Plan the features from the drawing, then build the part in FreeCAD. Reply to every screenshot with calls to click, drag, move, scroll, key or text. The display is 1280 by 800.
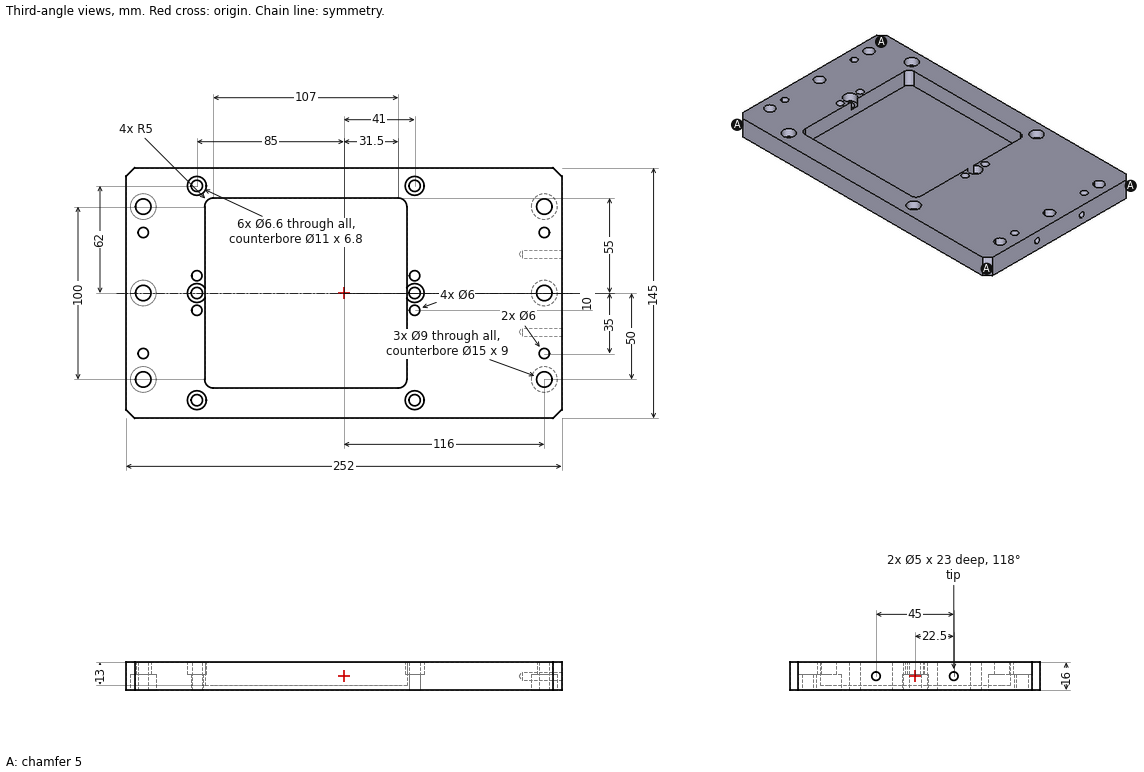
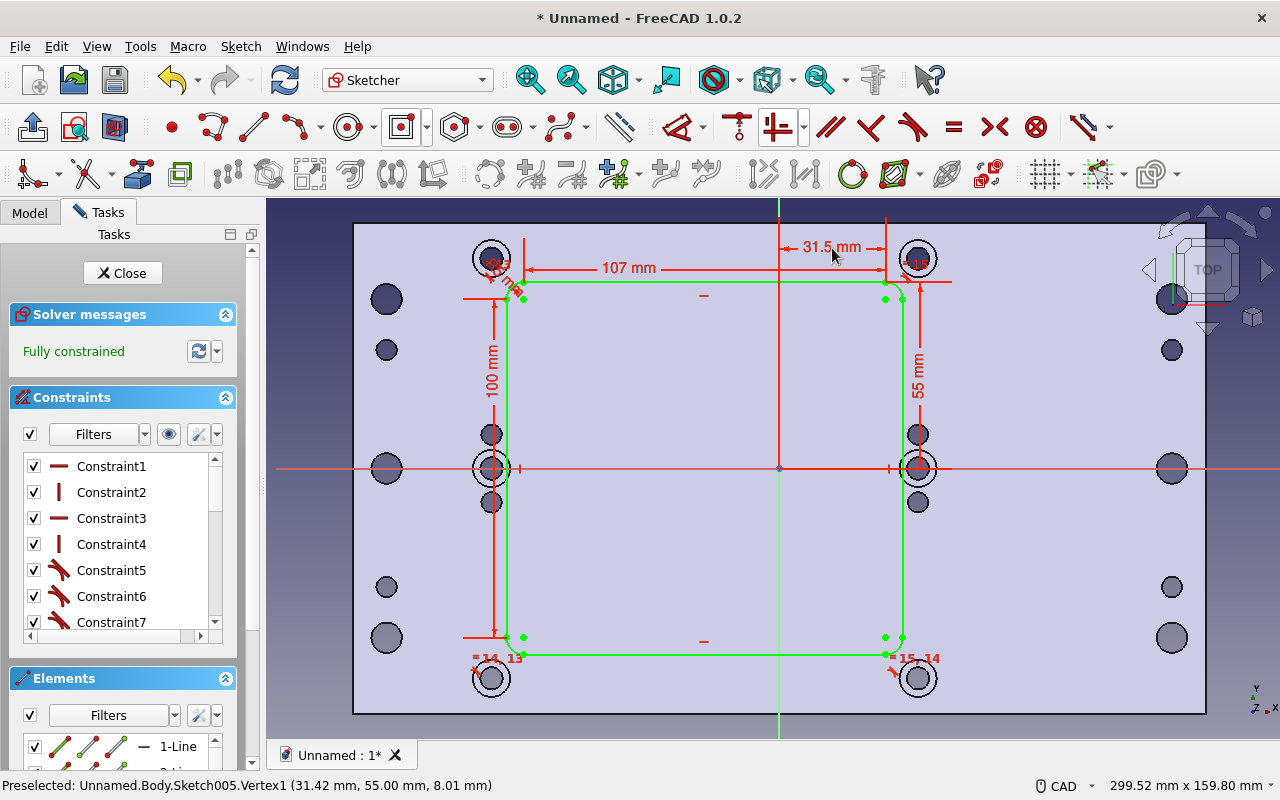
click(123, 273)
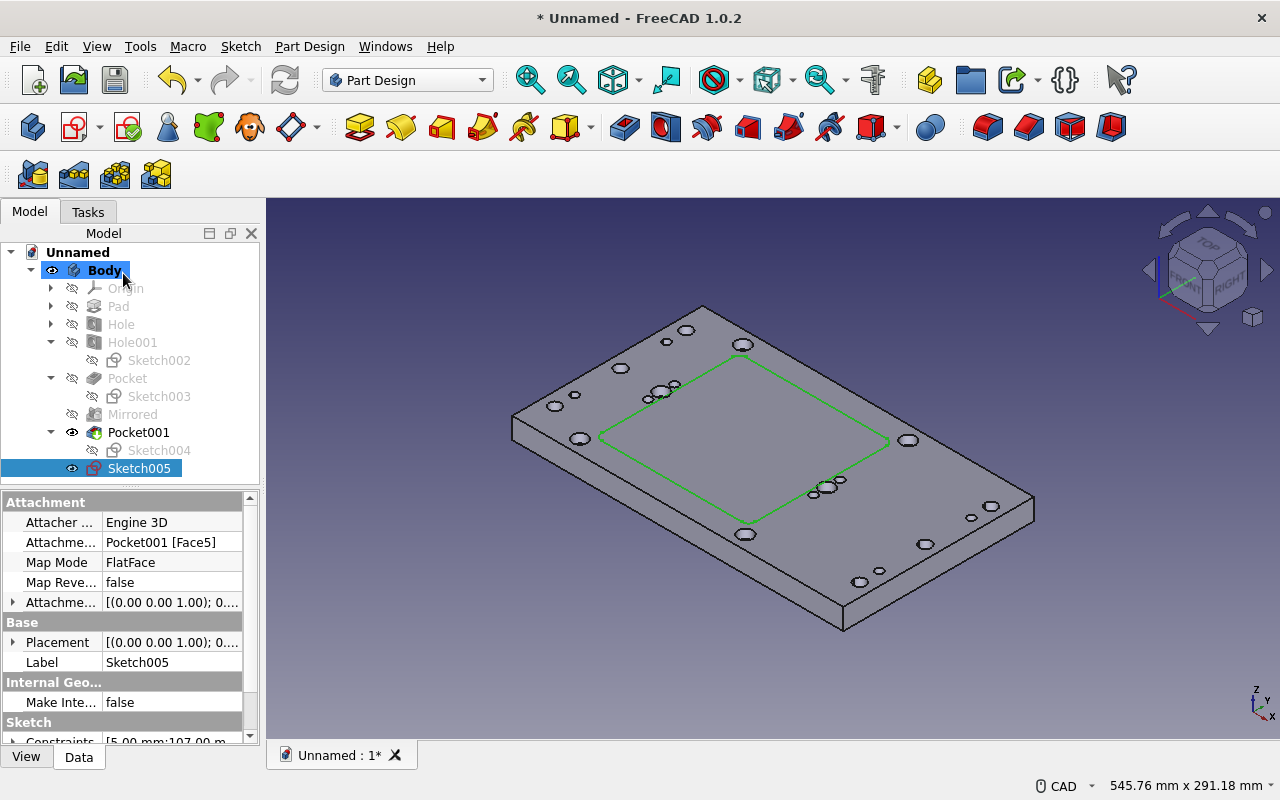
click(625, 128)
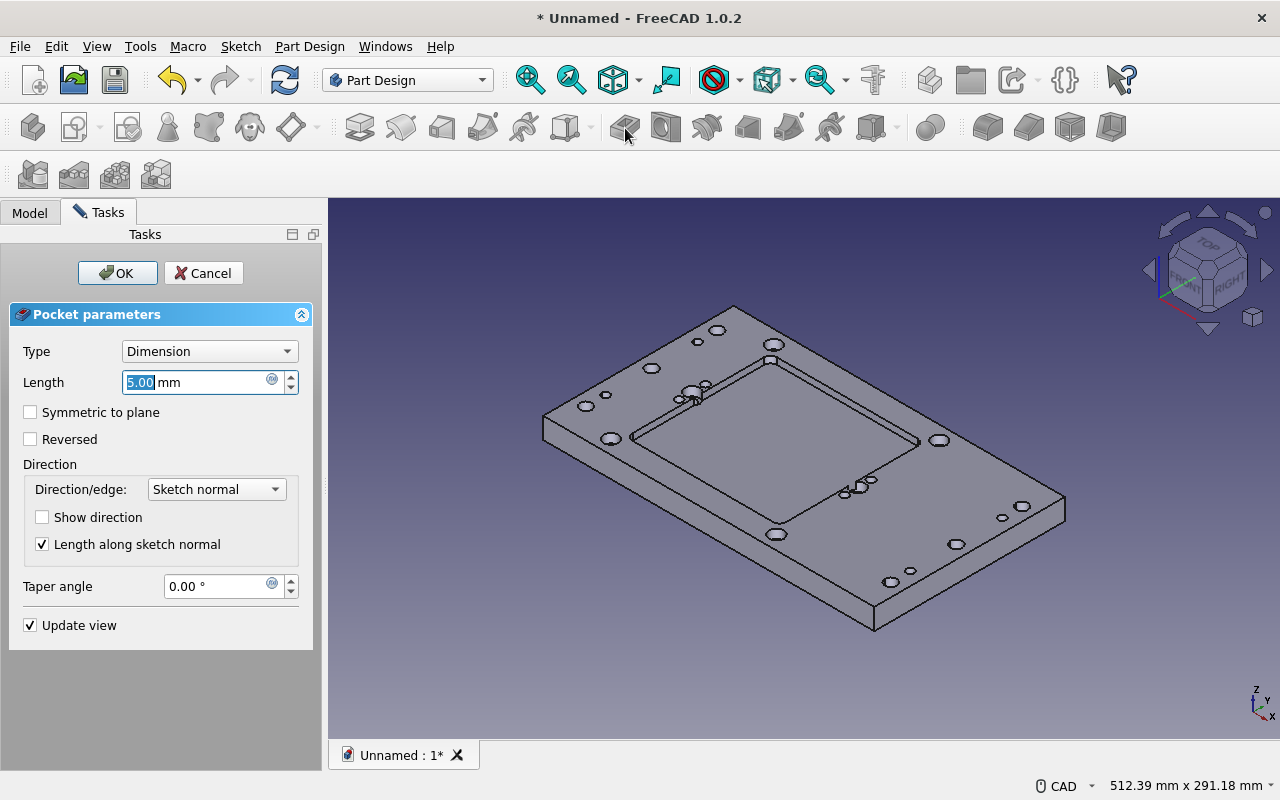
text(13)
key(Tab)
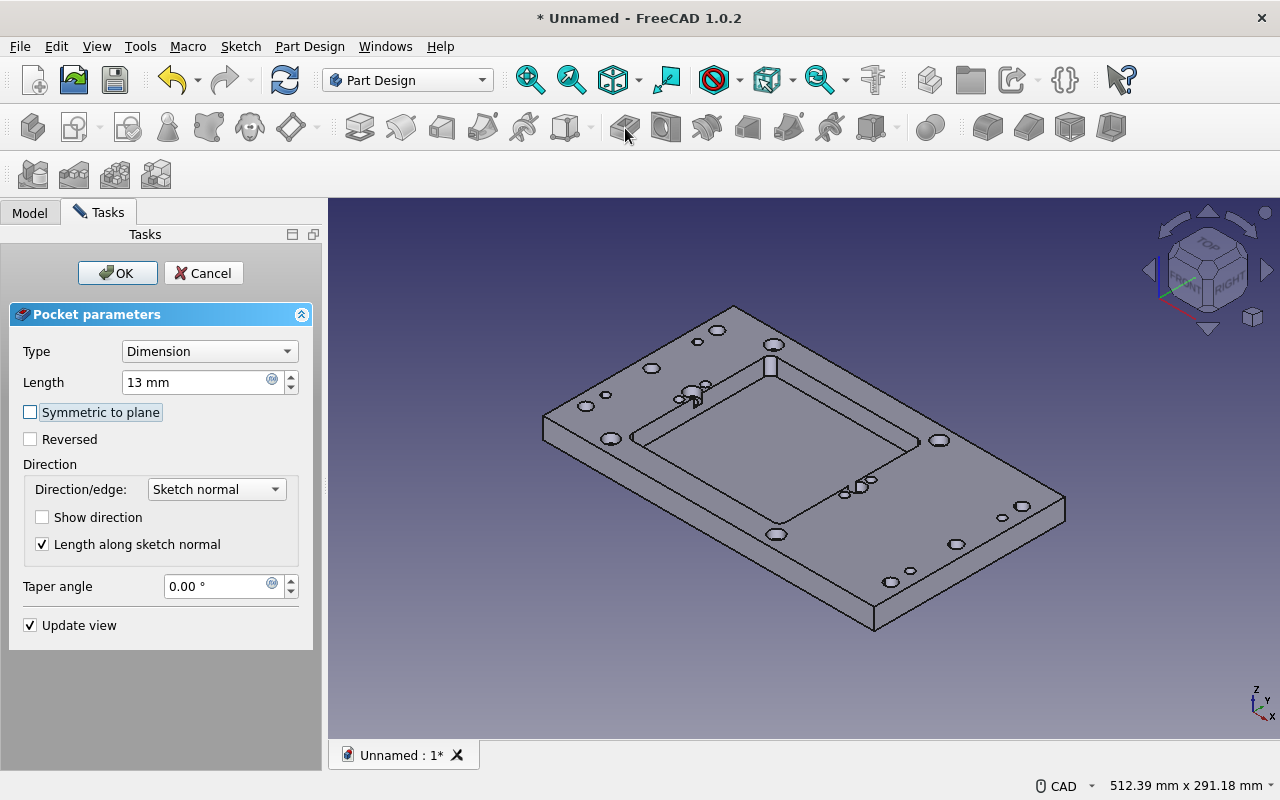
click(118, 273)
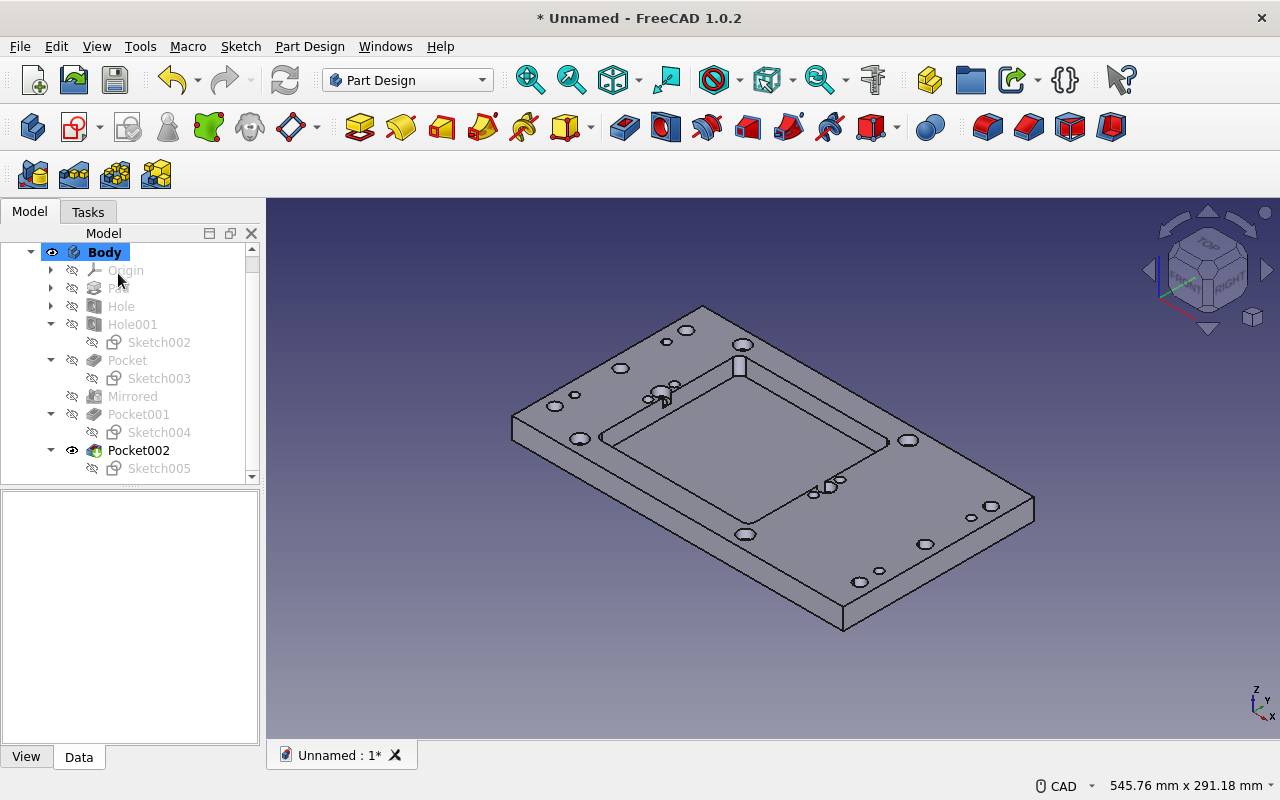
click(843, 618)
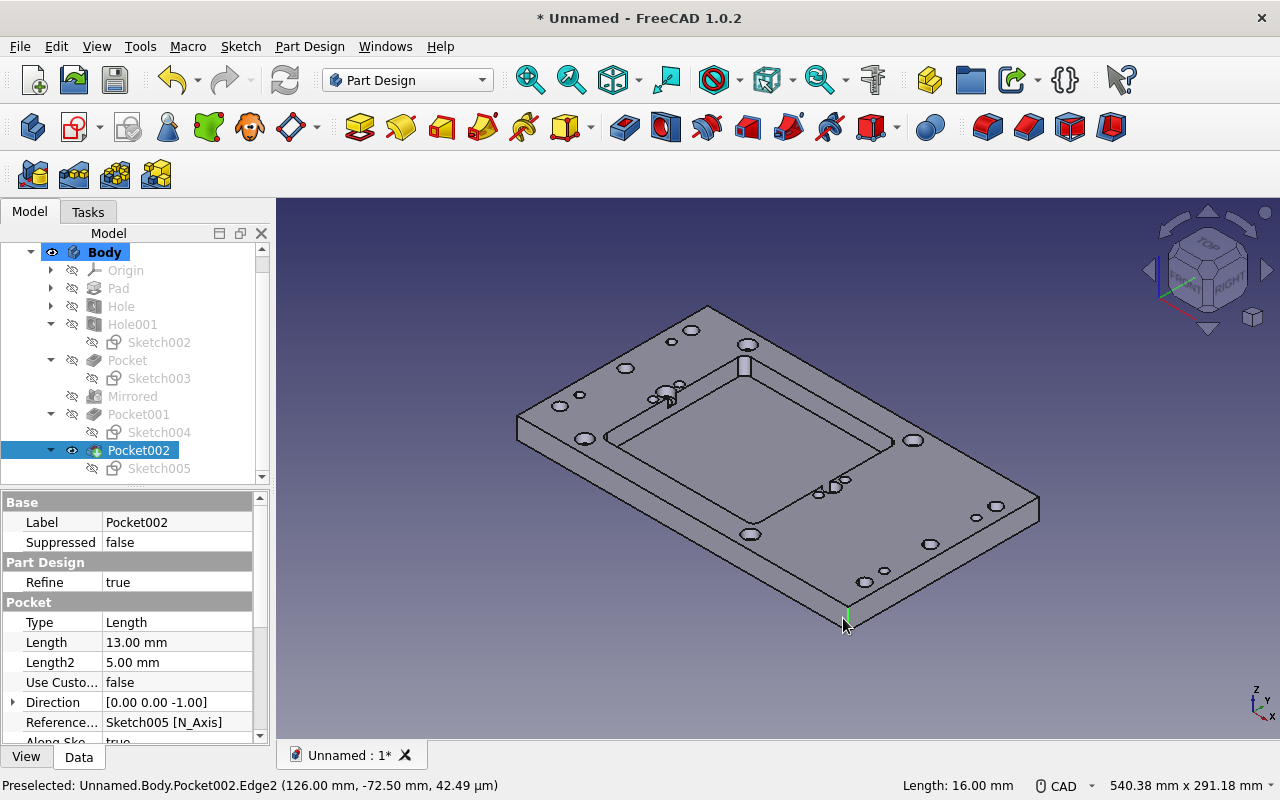
key(2)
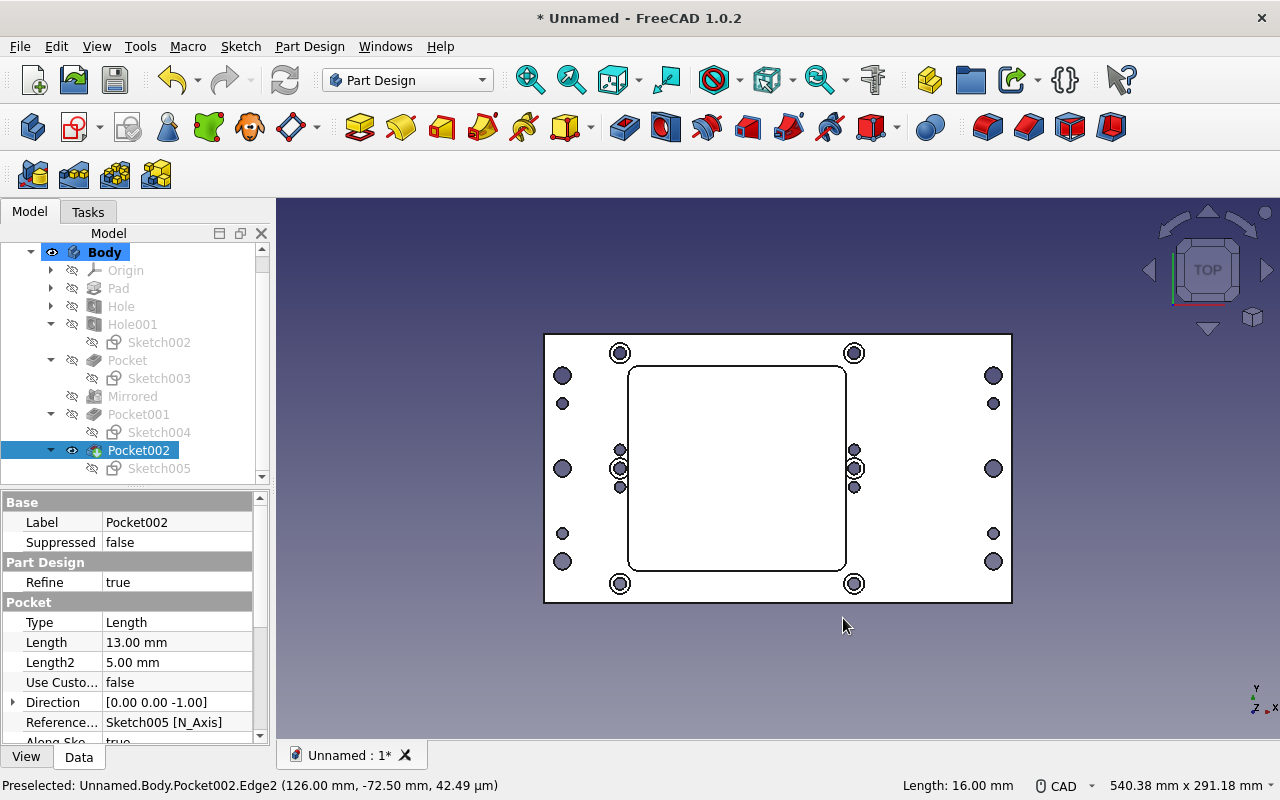
key(0)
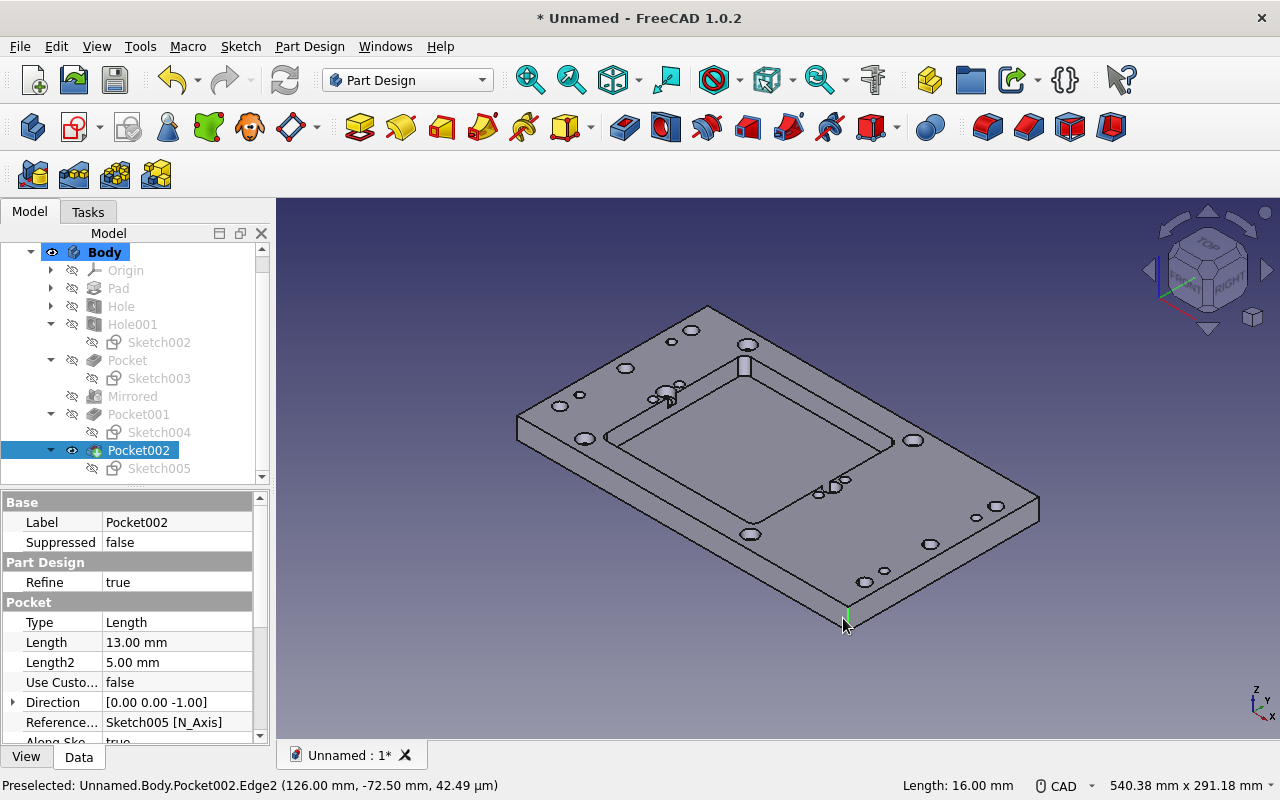
key(1)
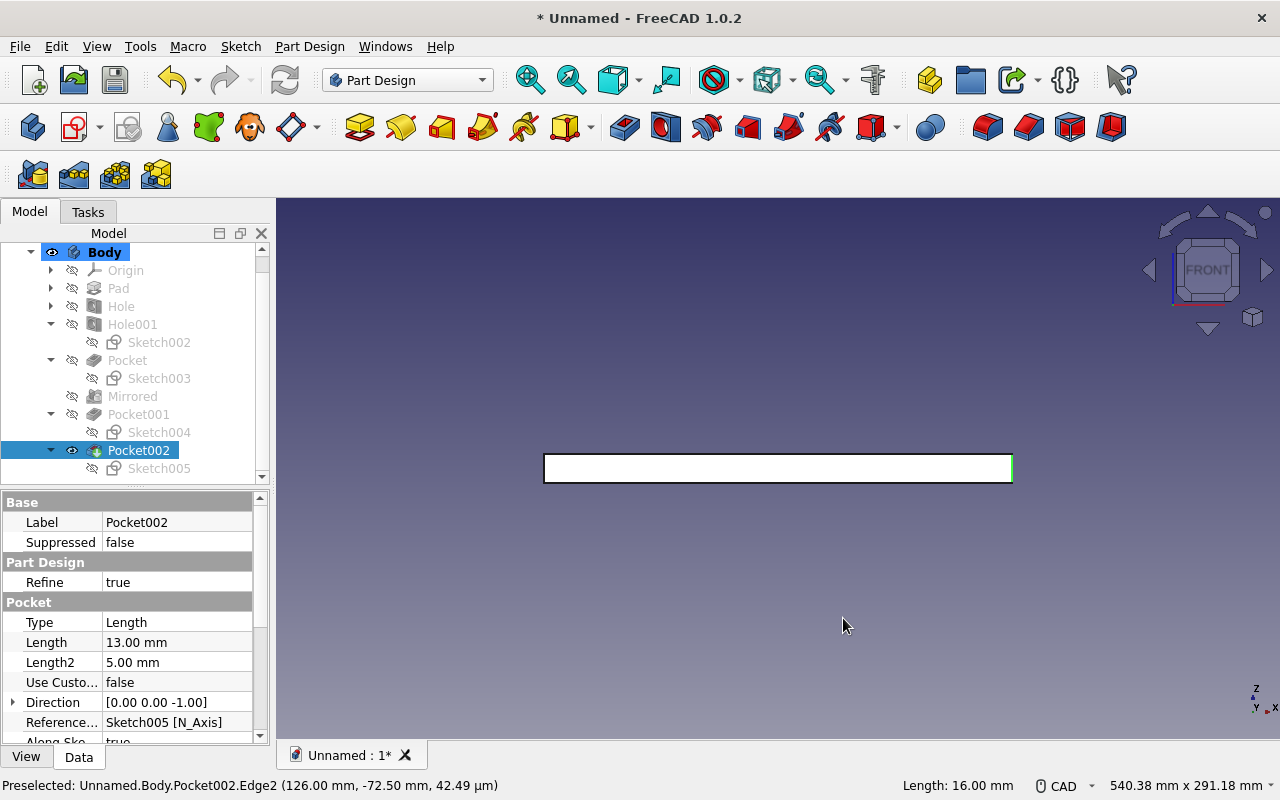
click(544, 467, ctrl)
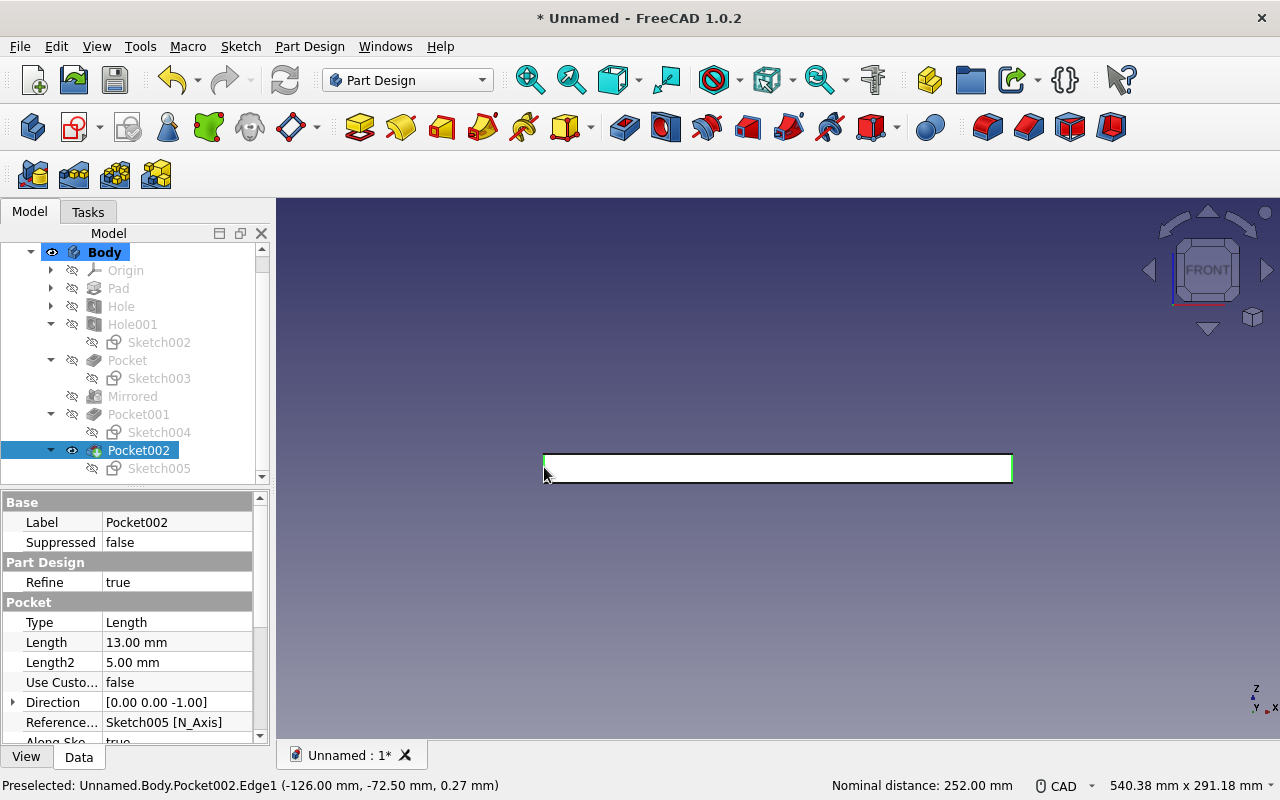
key(3)